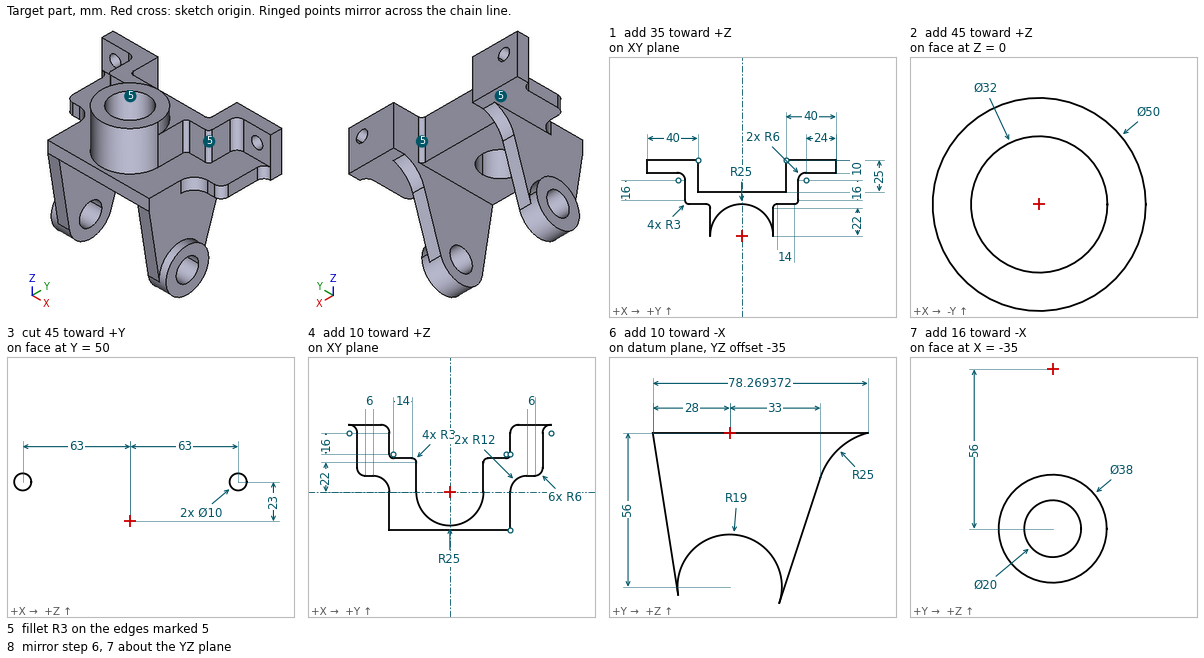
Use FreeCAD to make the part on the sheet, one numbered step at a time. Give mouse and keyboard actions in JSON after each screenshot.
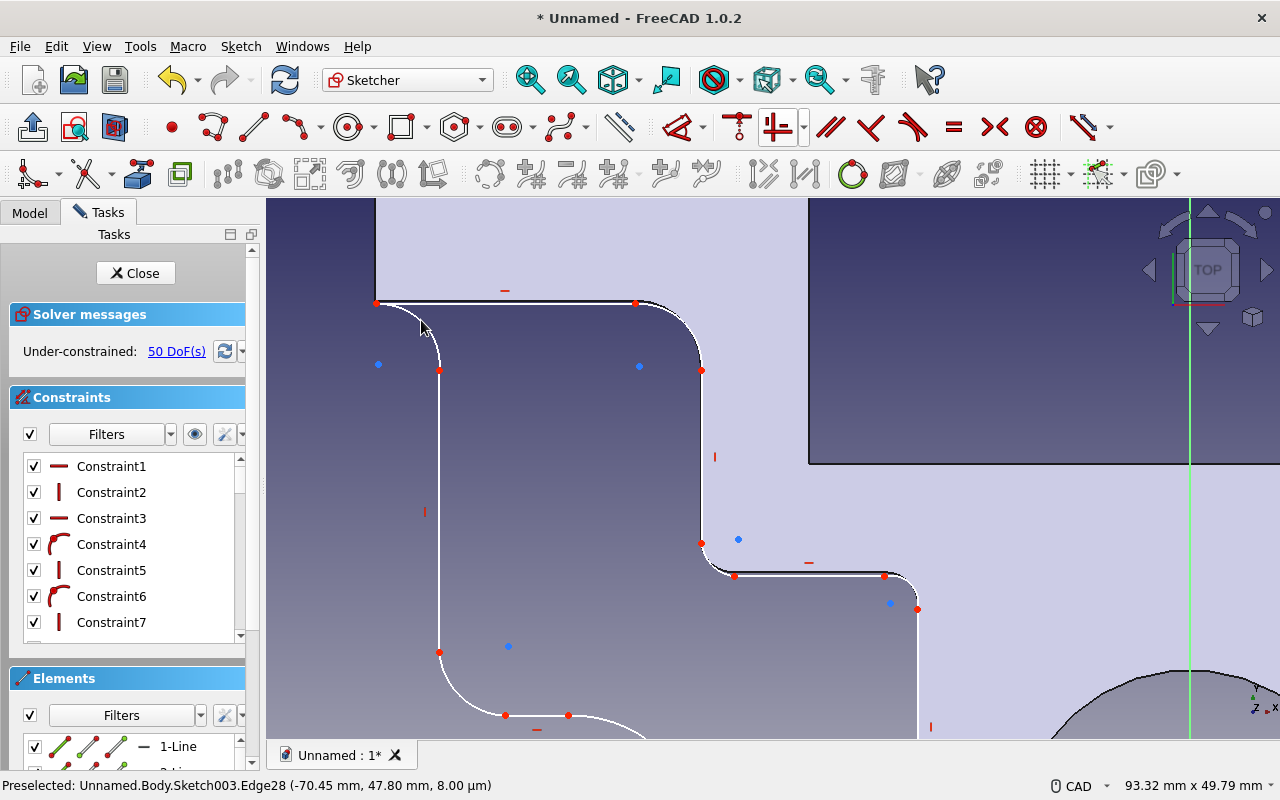
{"action": "left_click", "coordinate": [454, 304]}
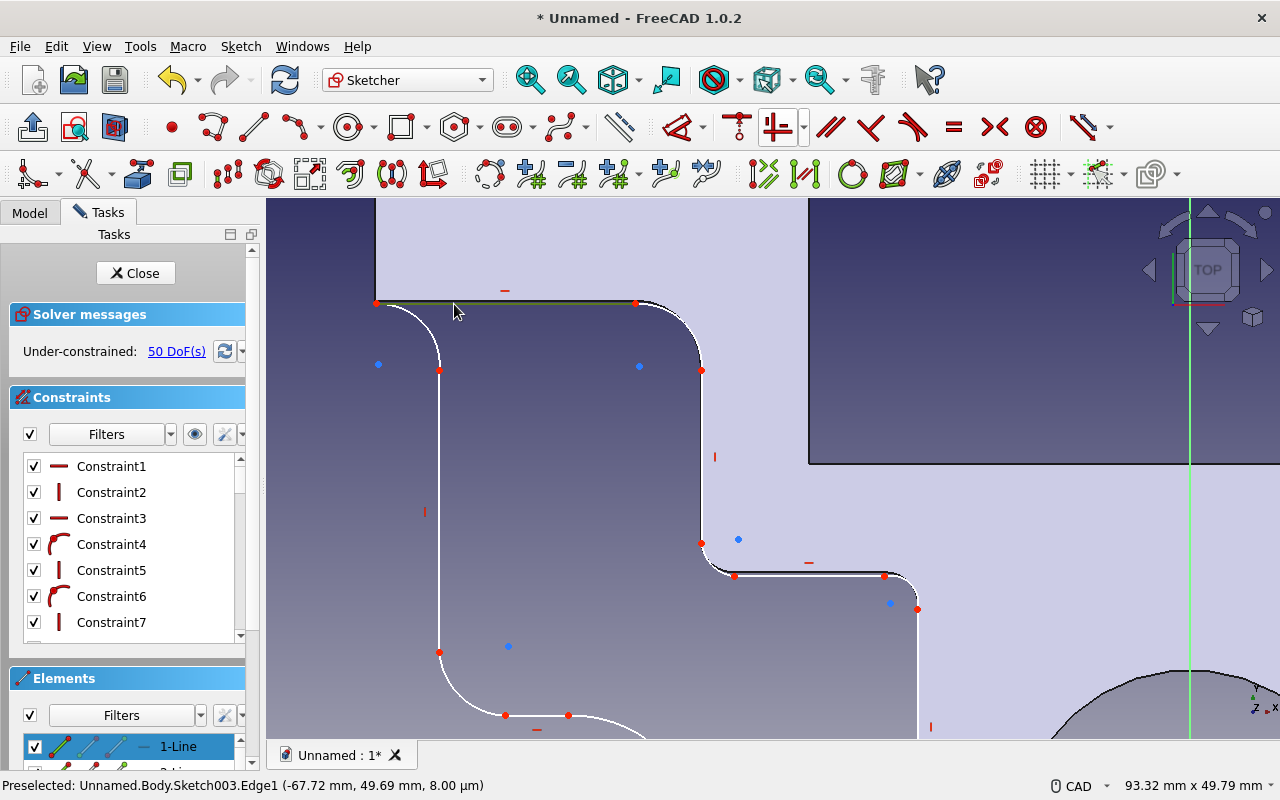
{"action": "left_click", "coordinate": [696, 339]}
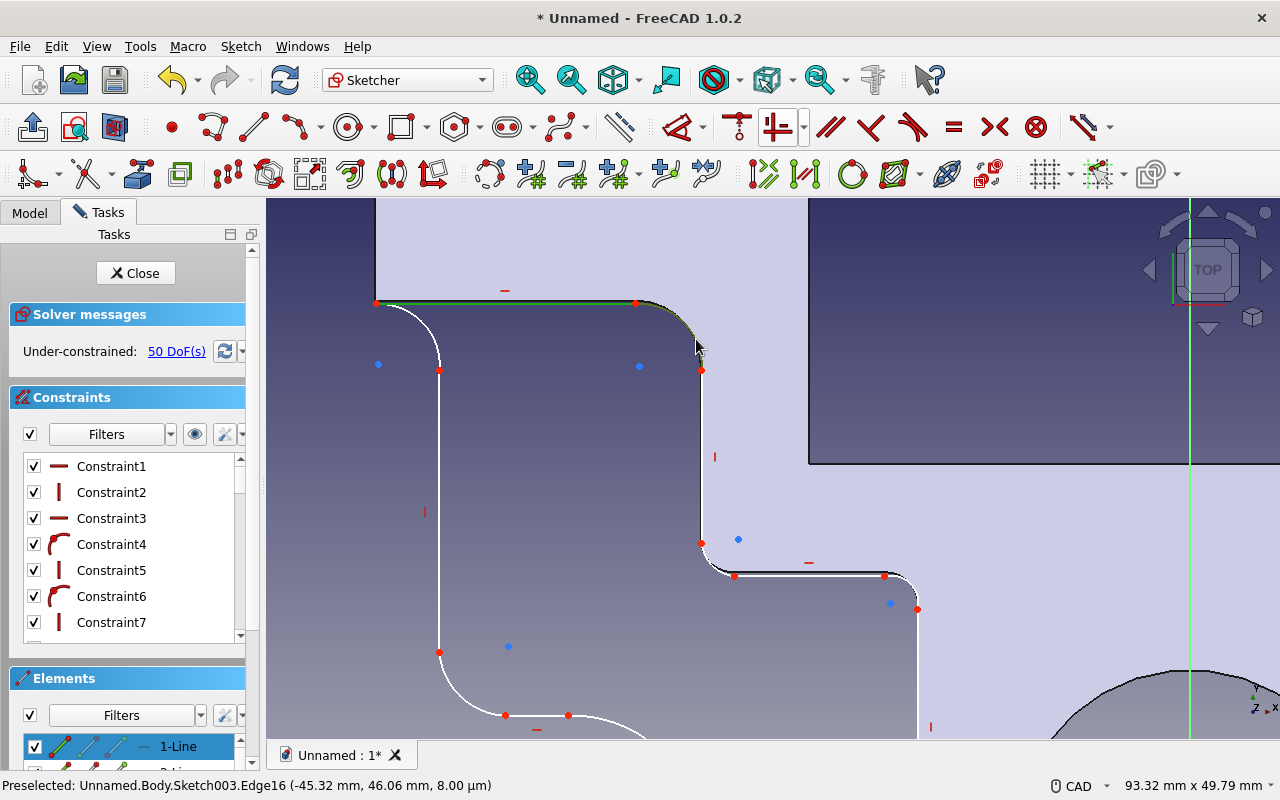
{"action": "left_click", "coordinate": [913, 128]}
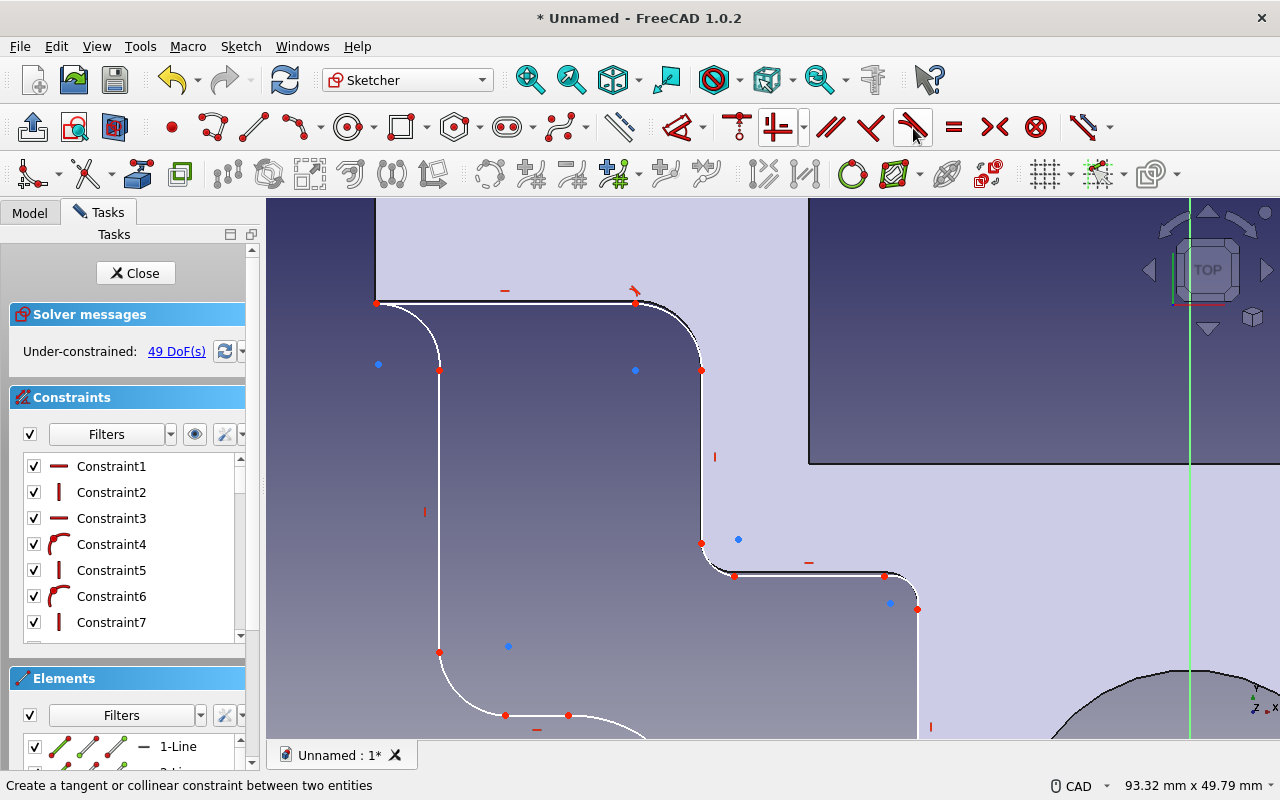
{"action": "left_click", "coordinate": [454, 304]}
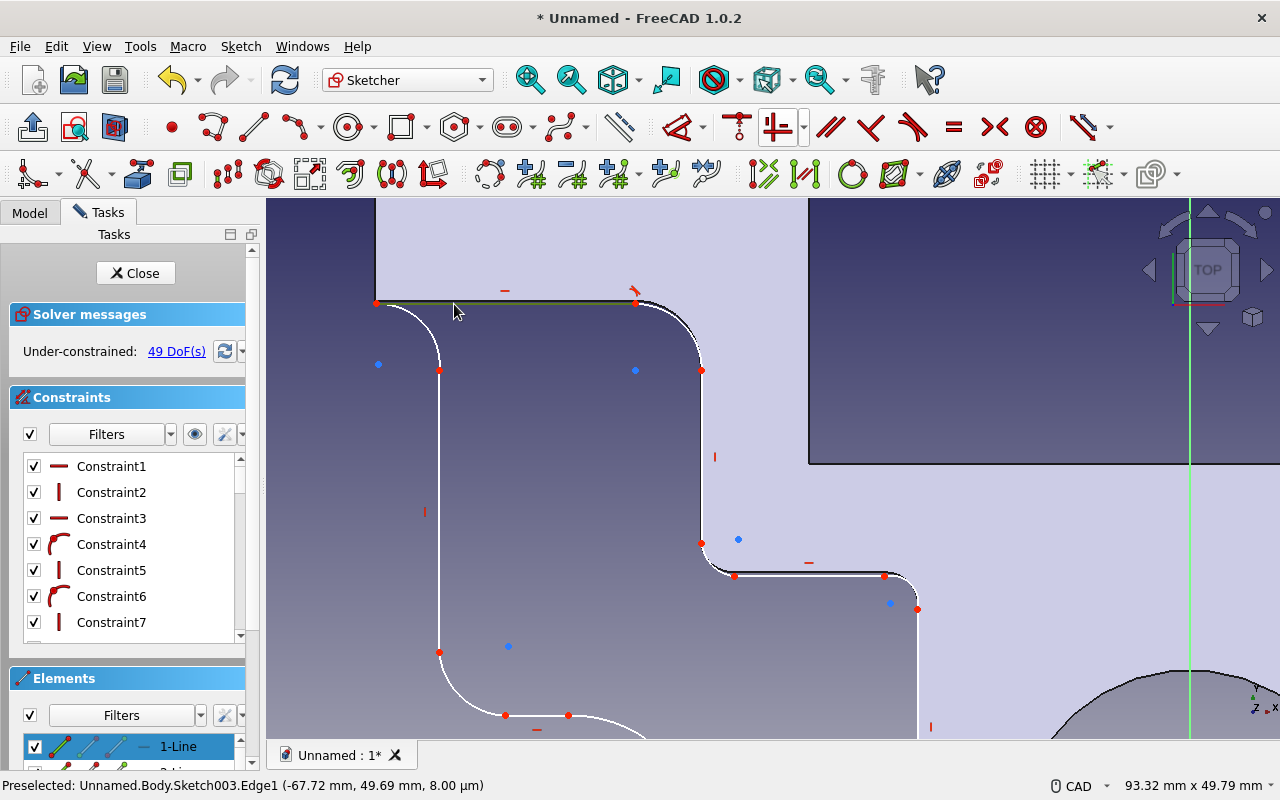
{"action": "left_click", "coordinate": [434, 340]}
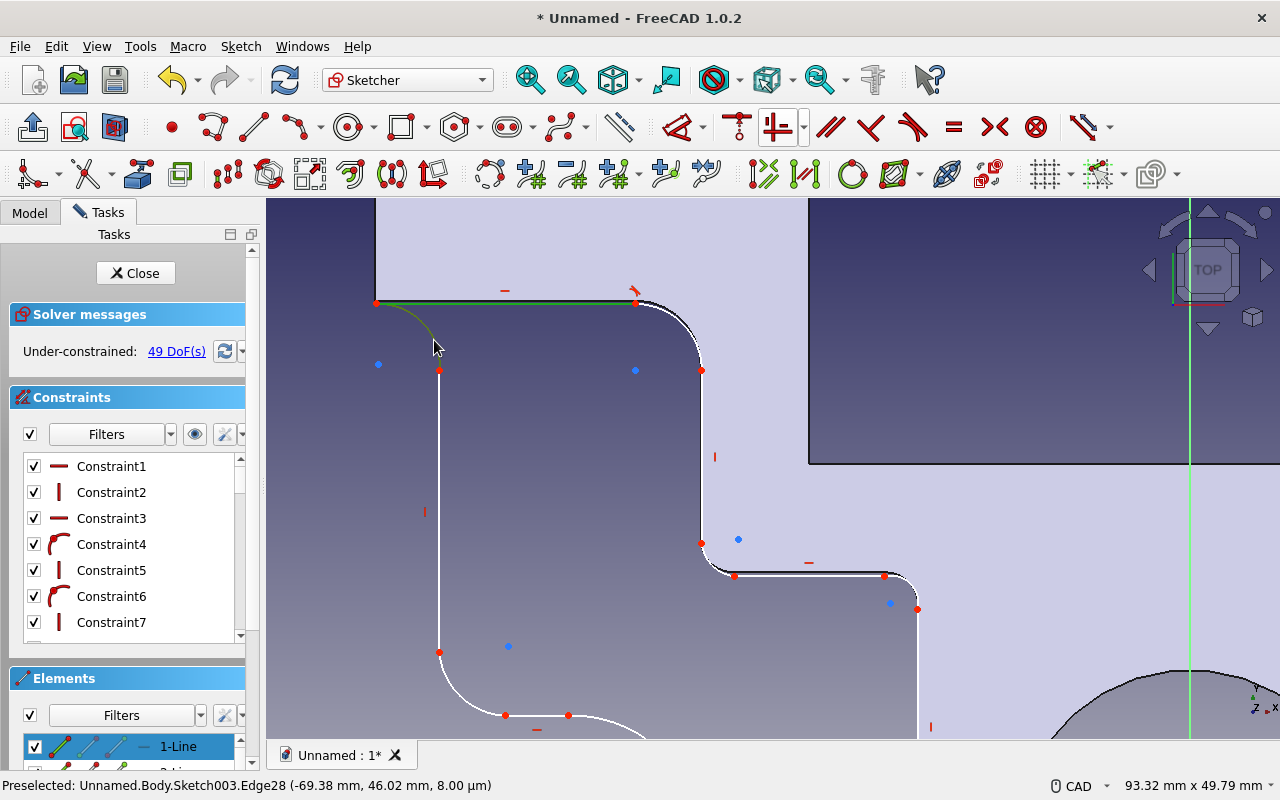
{"action": "left_click", "coordinate": [913, 128]}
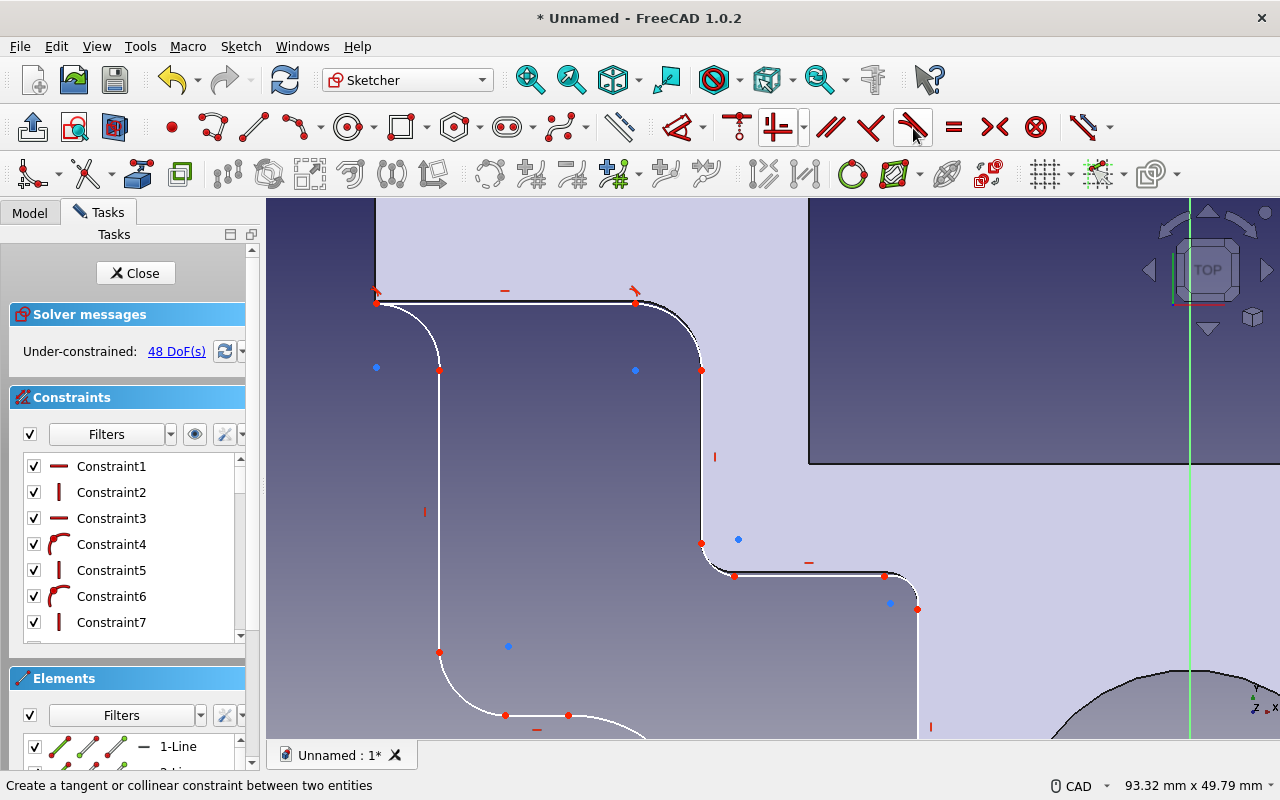
{"action": "left_click", "coordinate": [702, 422]}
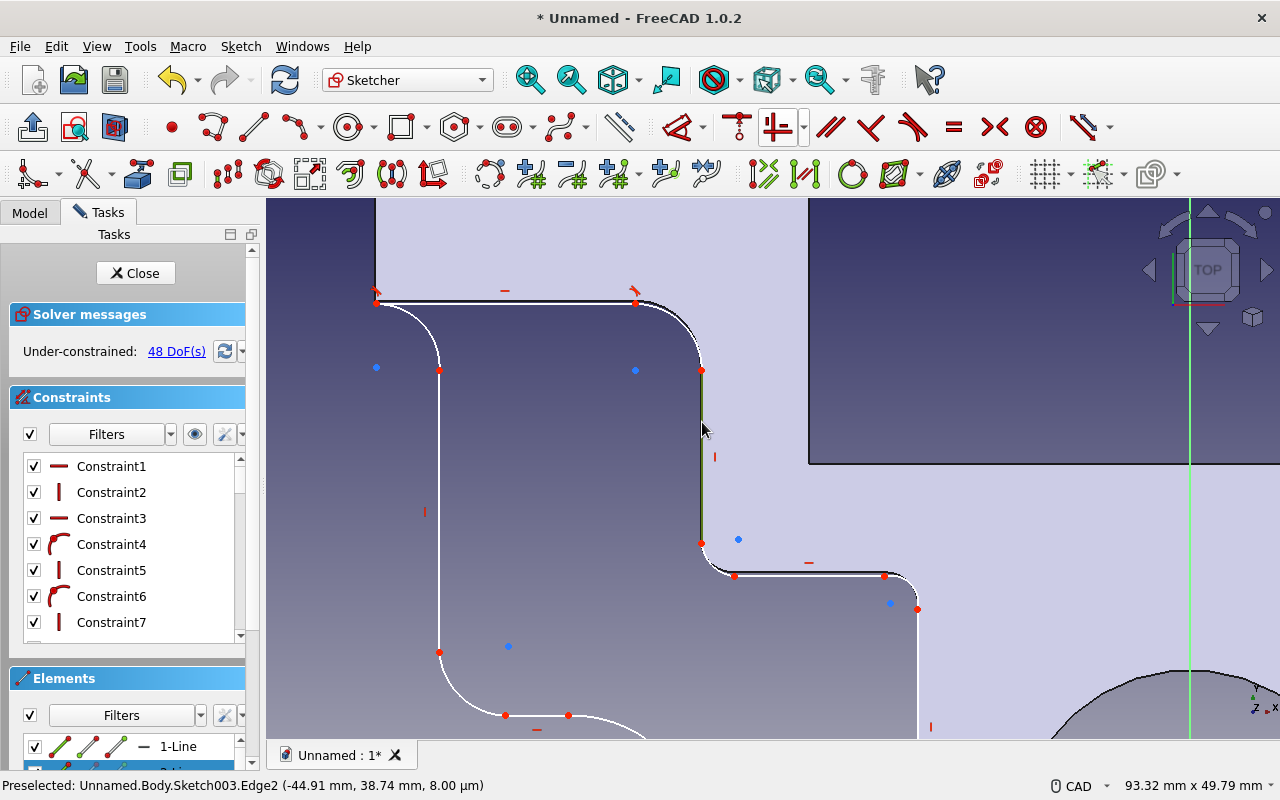
{"action": "left_click", "coordinate": [695, 340]}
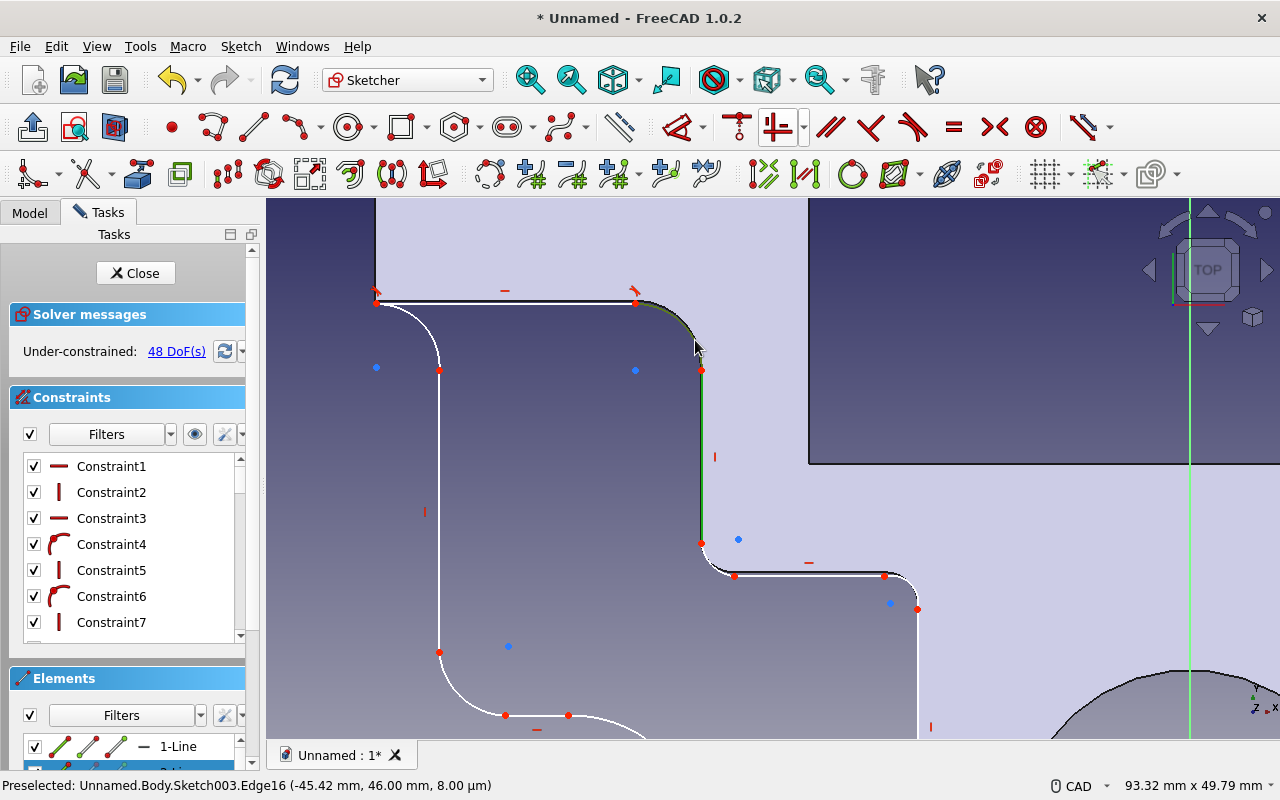
{"action": "left_click", "coordinate": [913, 128]}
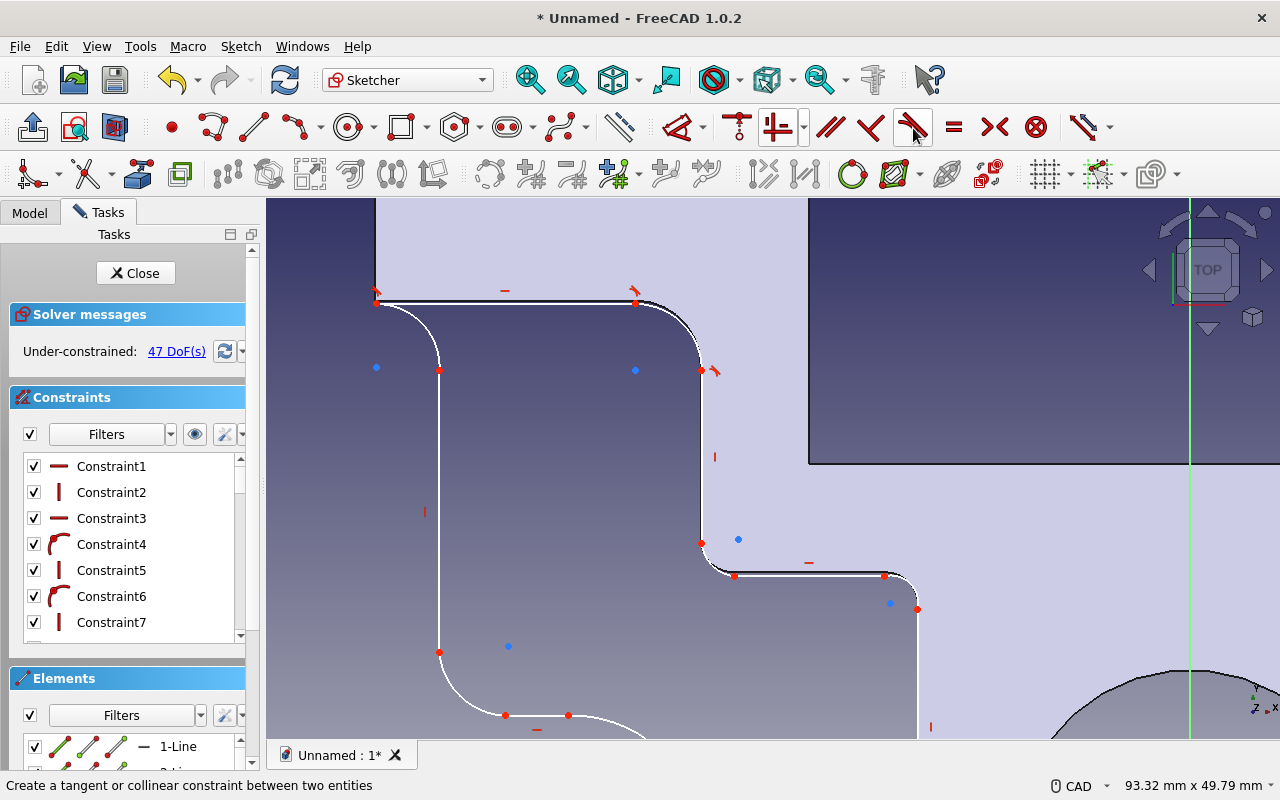
{"action": "left_click", "coordinate": [702, 422]}